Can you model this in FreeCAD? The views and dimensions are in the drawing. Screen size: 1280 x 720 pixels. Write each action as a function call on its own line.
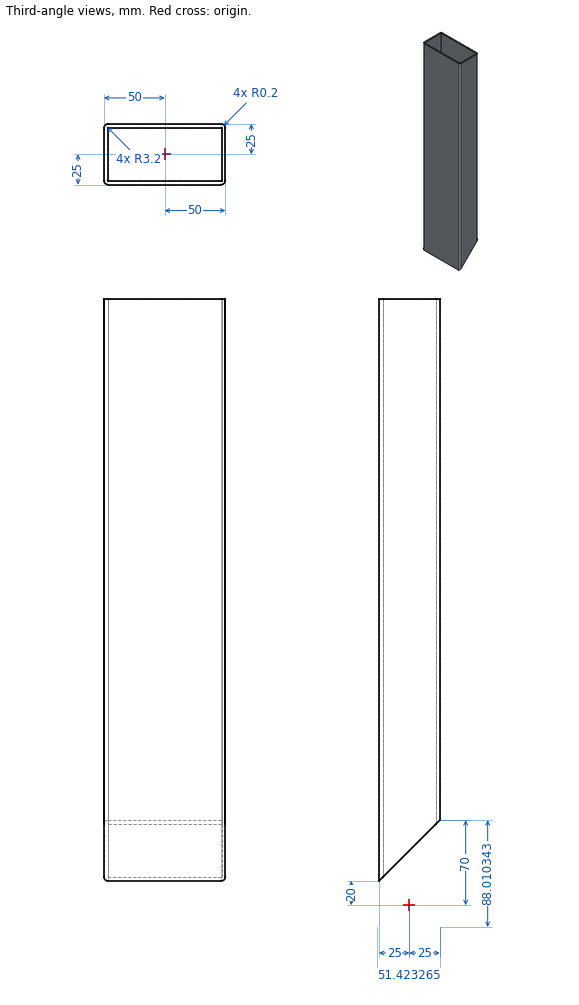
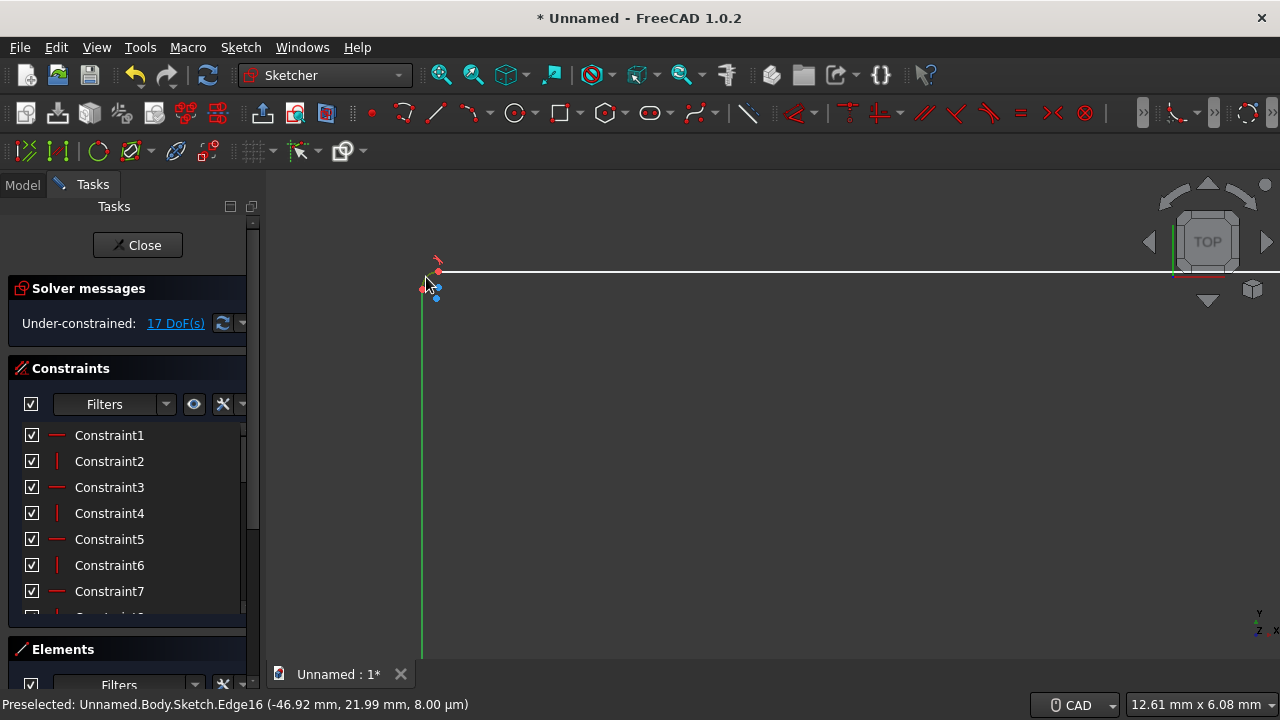
click(990, 114)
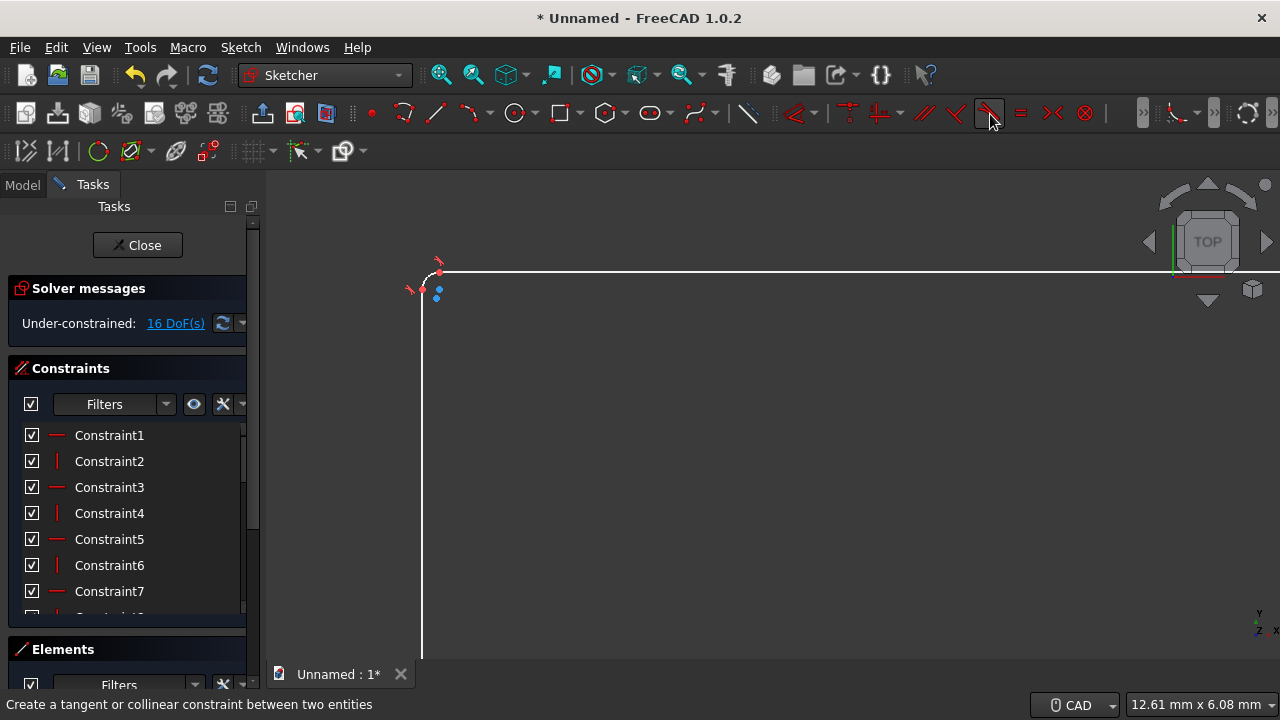
scroll(424, 284, down, 13)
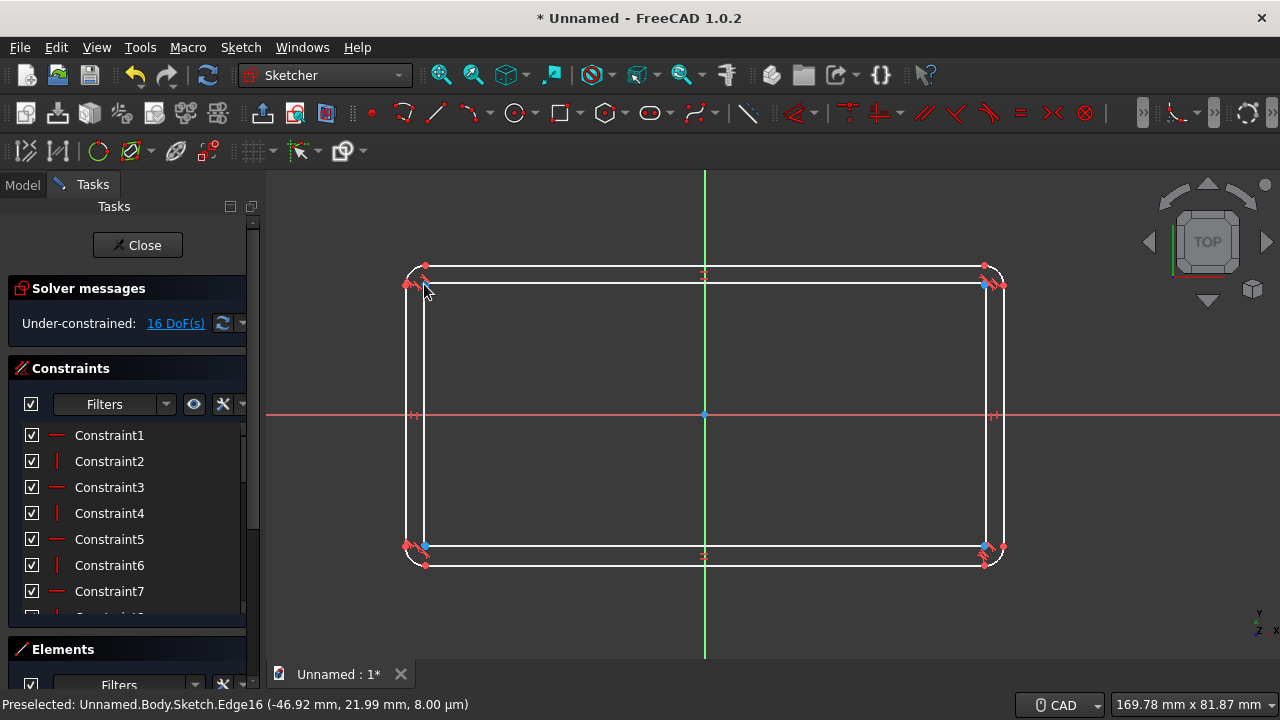
scroll(1002, 277, up, 3)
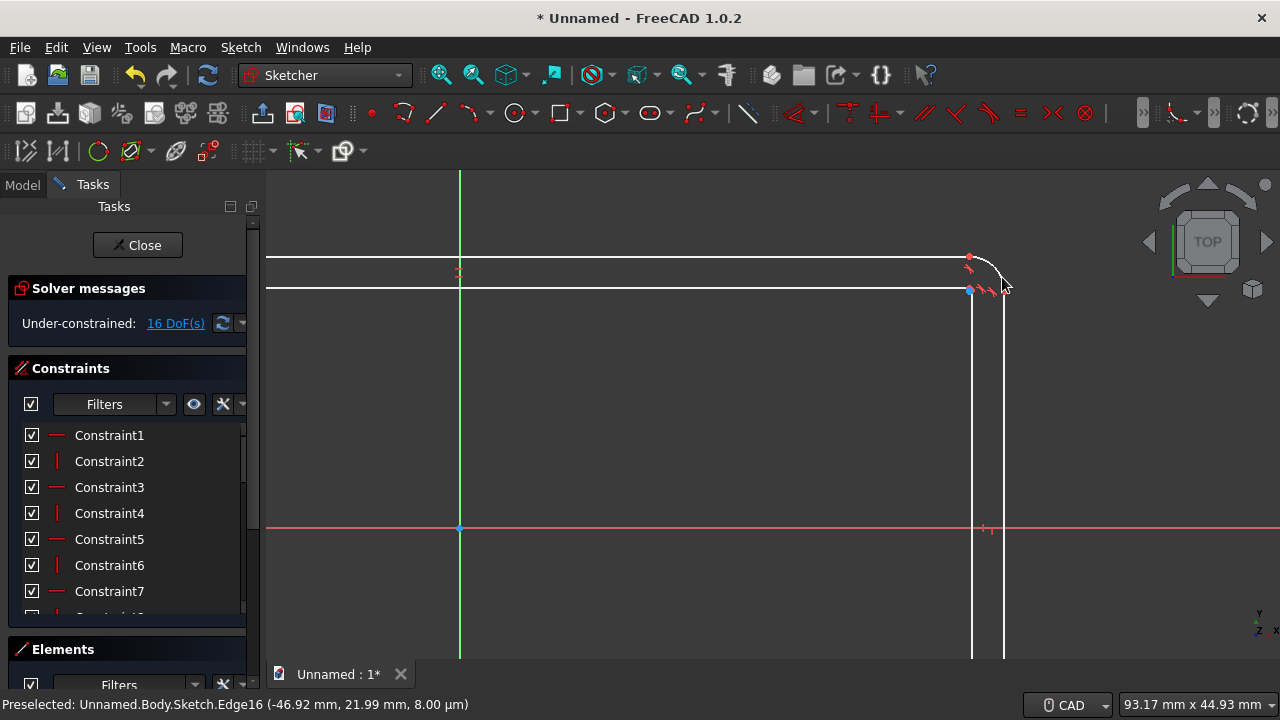
click(1001, 276)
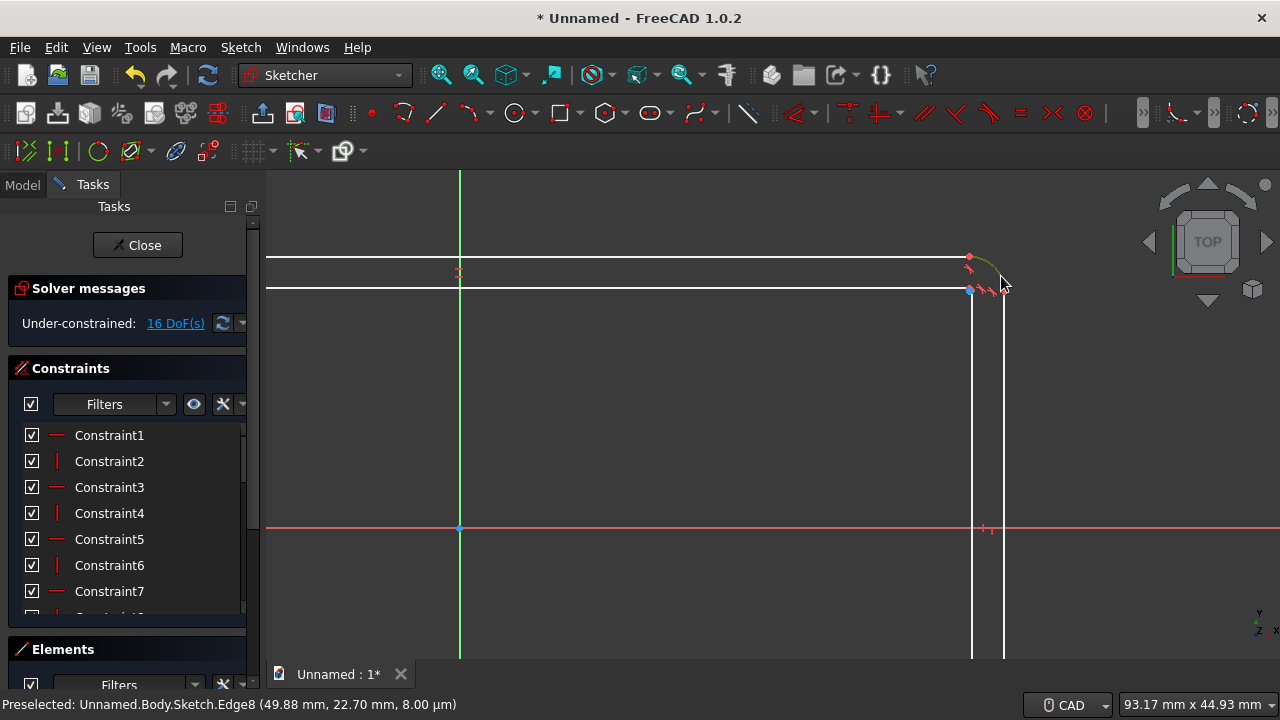
scroll(971, 289, up, 10)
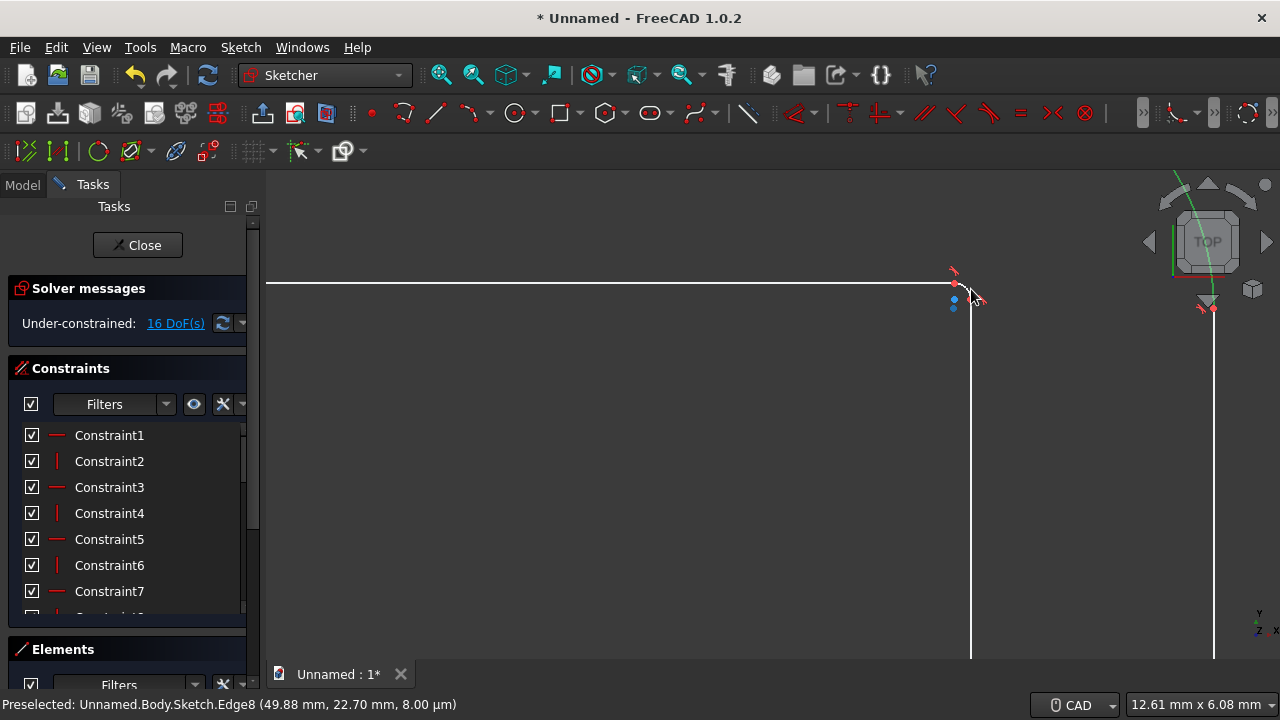
click(966, 288)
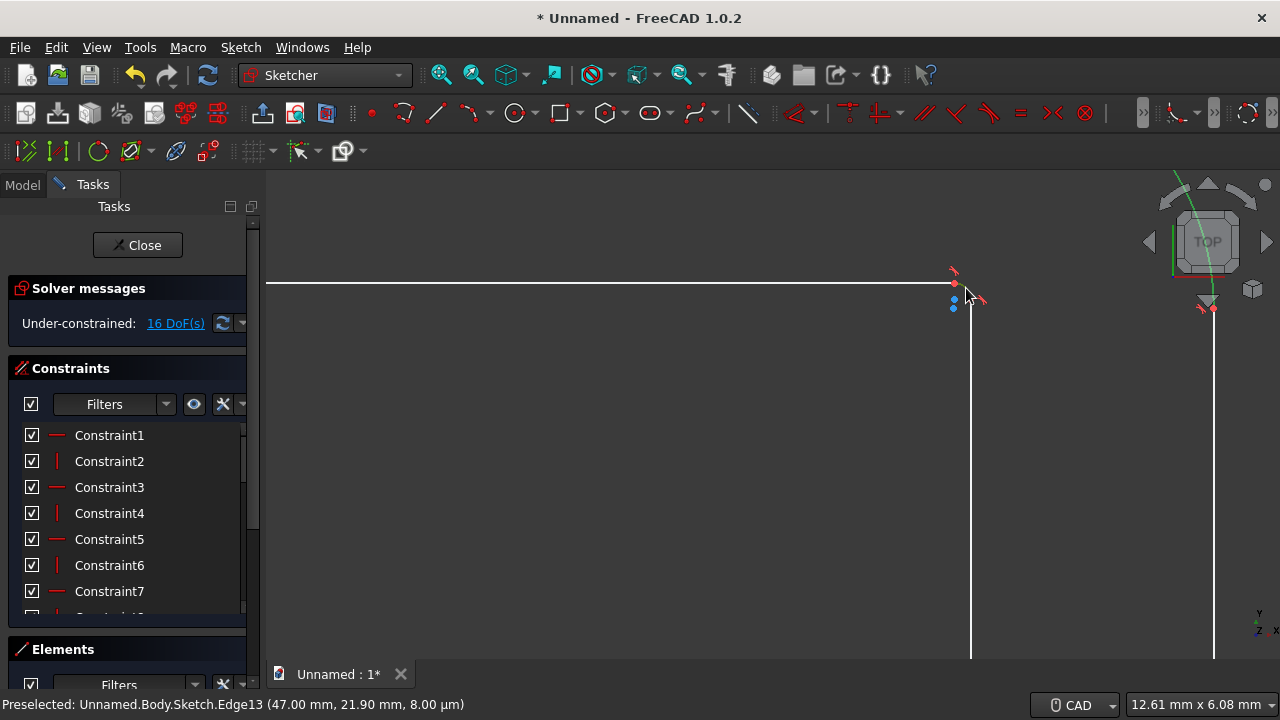
click(848, 114)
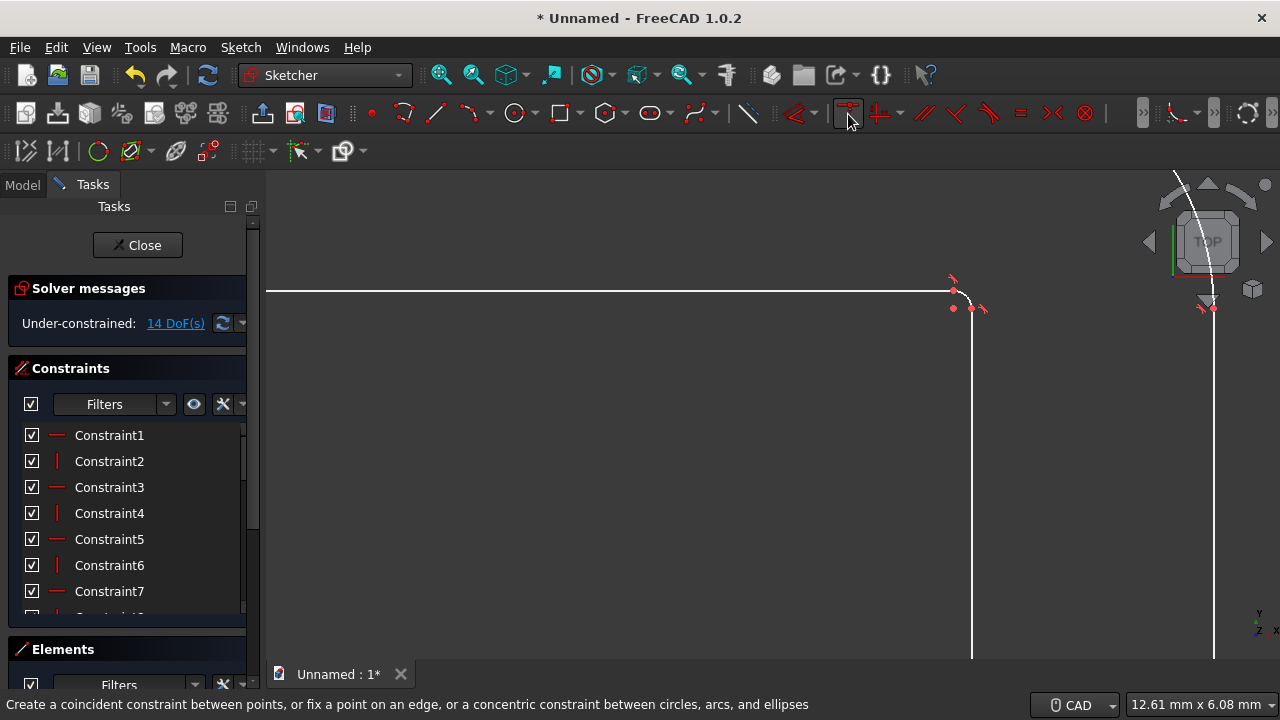
scroll(986, 283, down, 13)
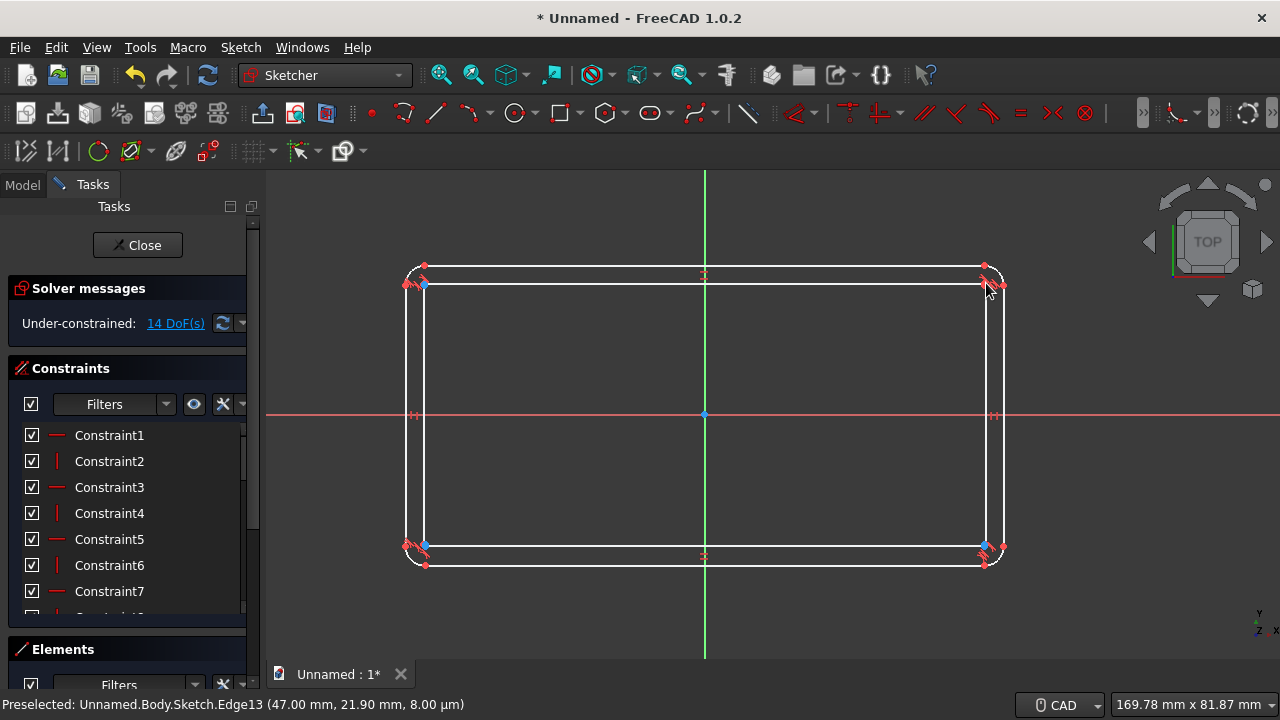
scroll(993, 564, up, 3)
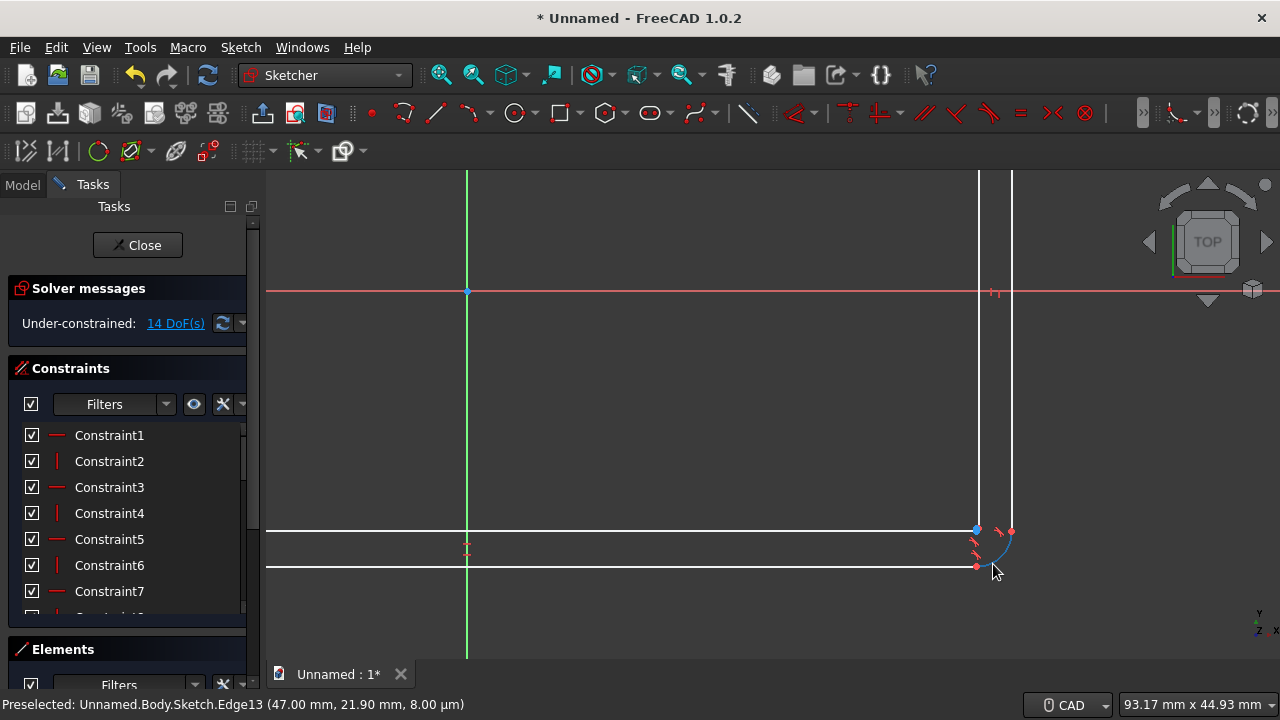
click(993, 563)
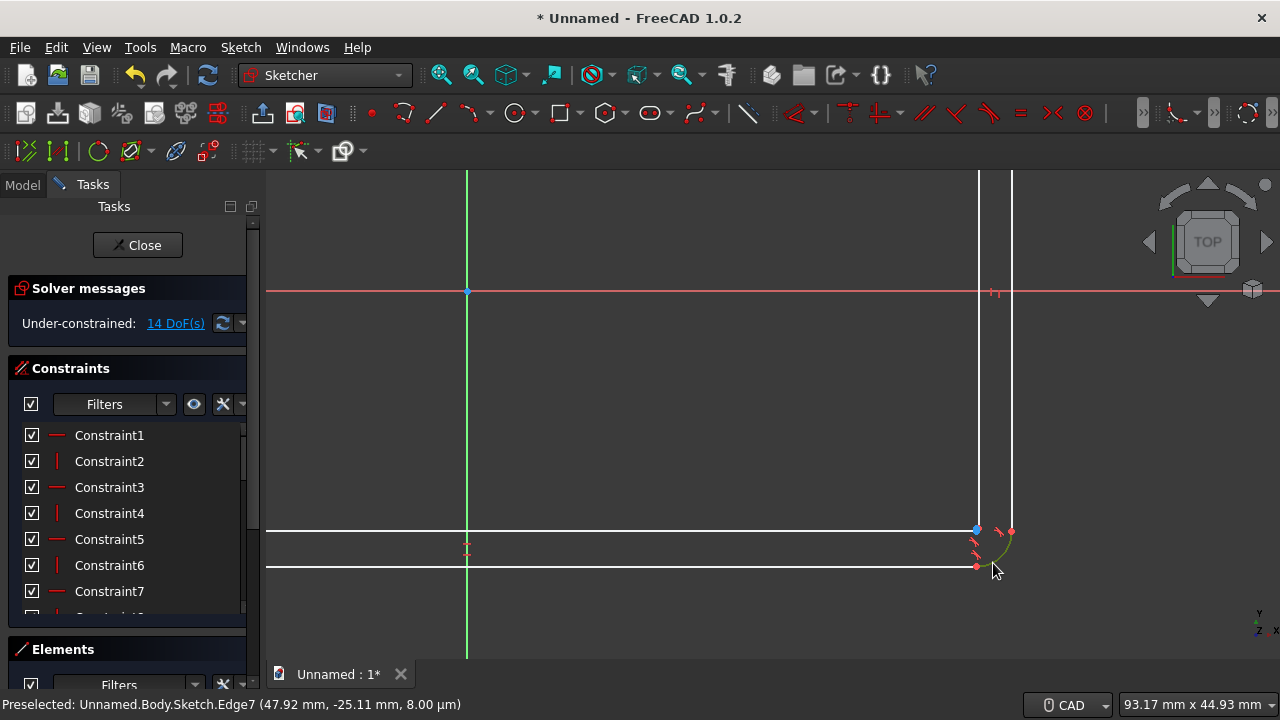
scroll(978, 530, up, 10)